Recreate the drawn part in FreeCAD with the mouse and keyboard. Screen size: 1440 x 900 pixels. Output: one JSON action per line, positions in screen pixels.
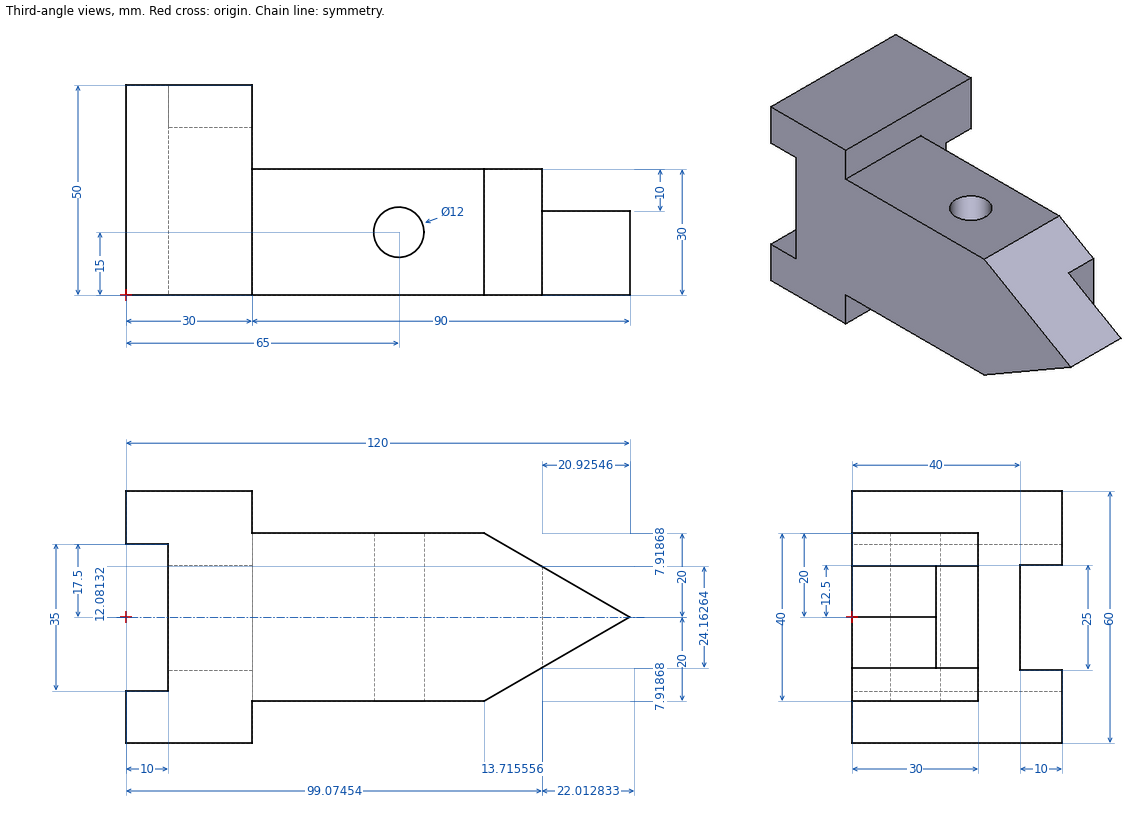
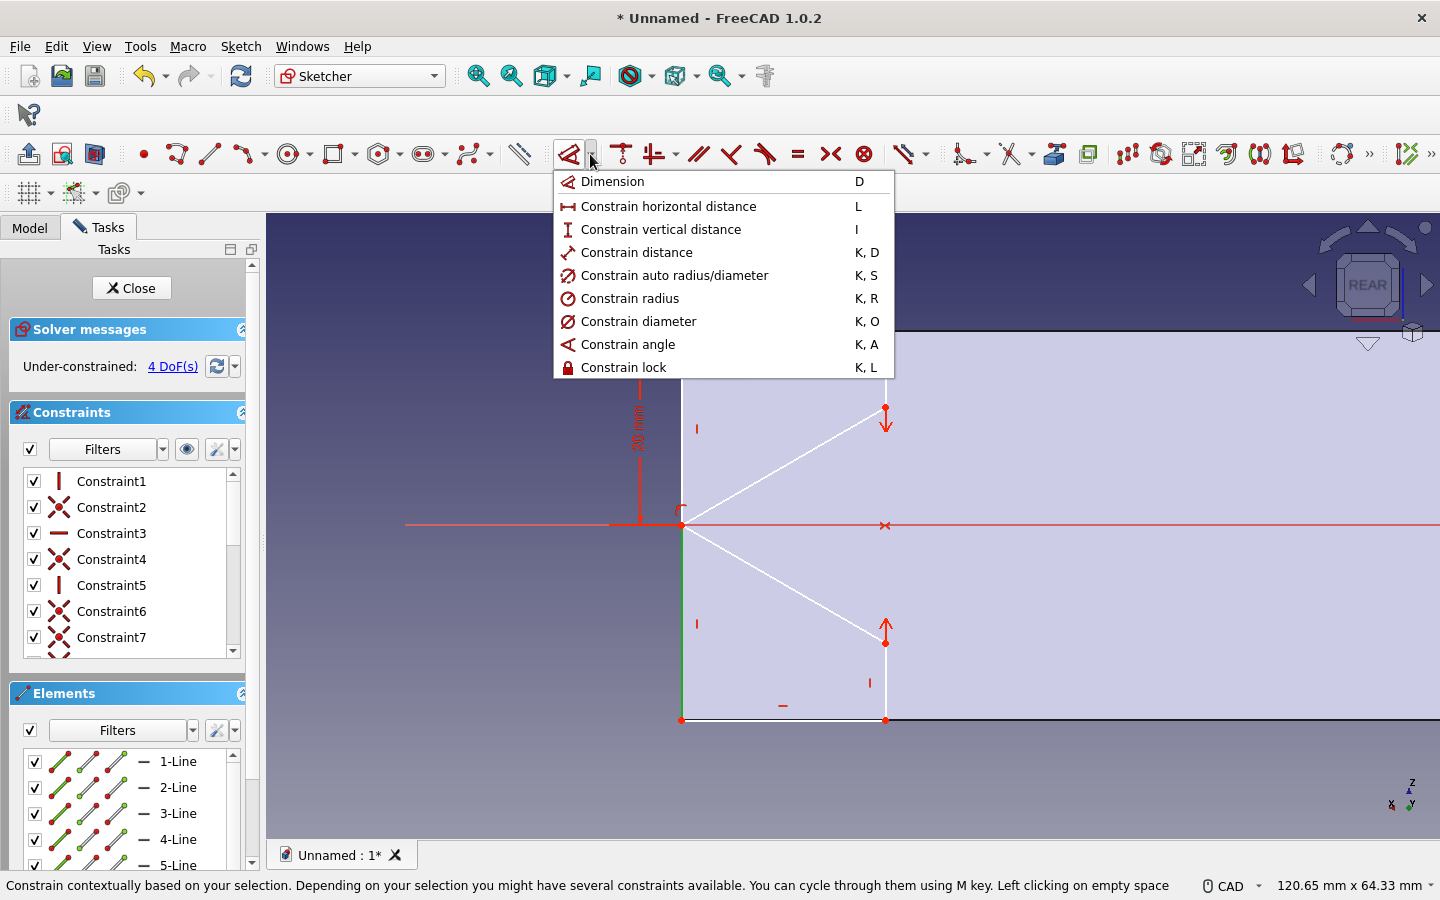
{"action": "left_click", "coordinate": [724, 230]}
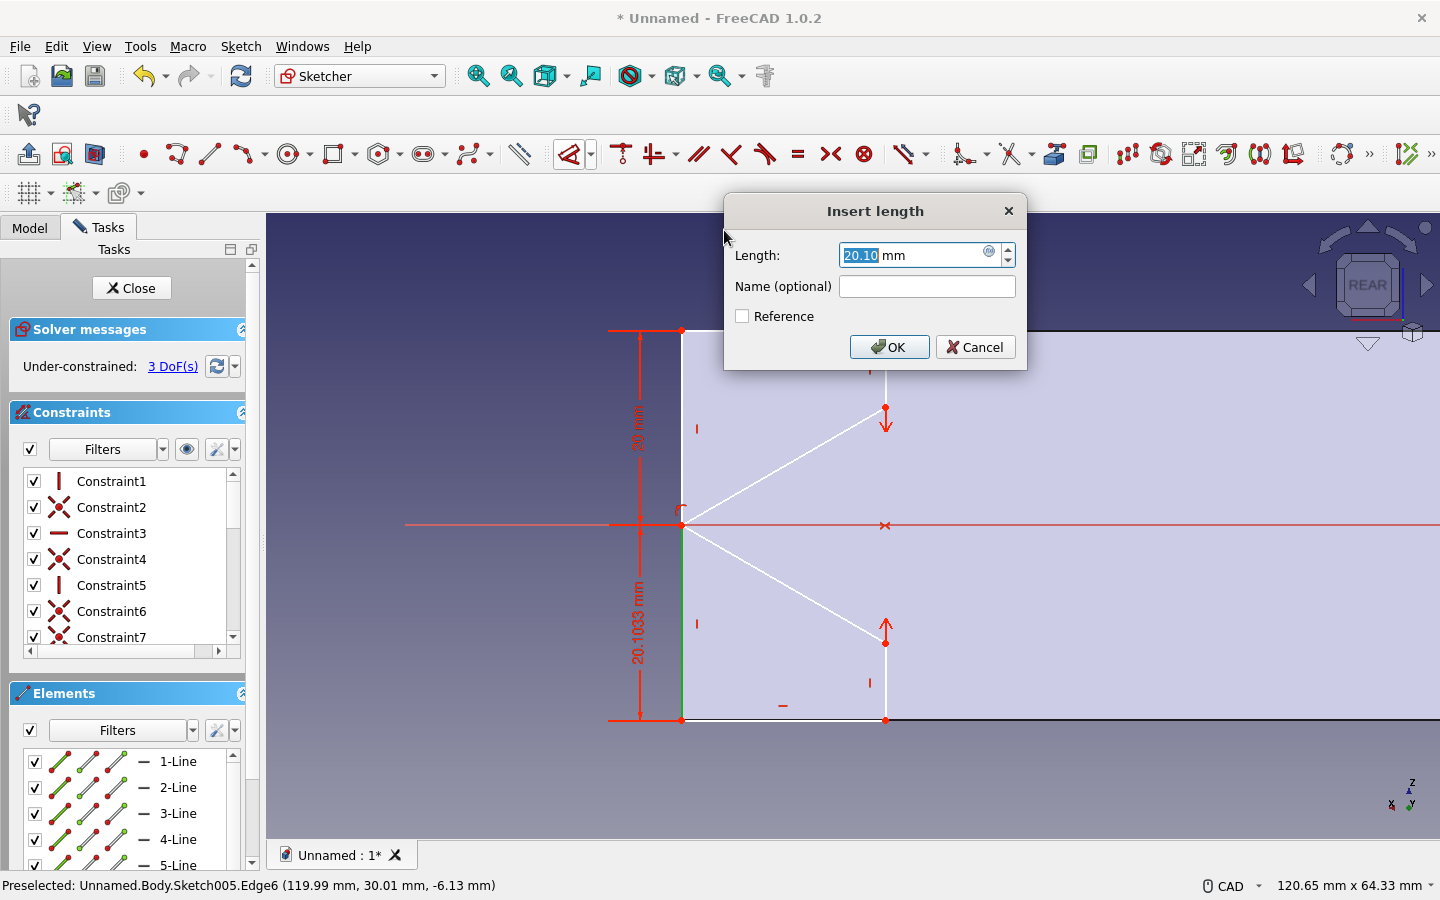
{"action": "type", "text": "20"}
{"action": "key", "text": "Return"}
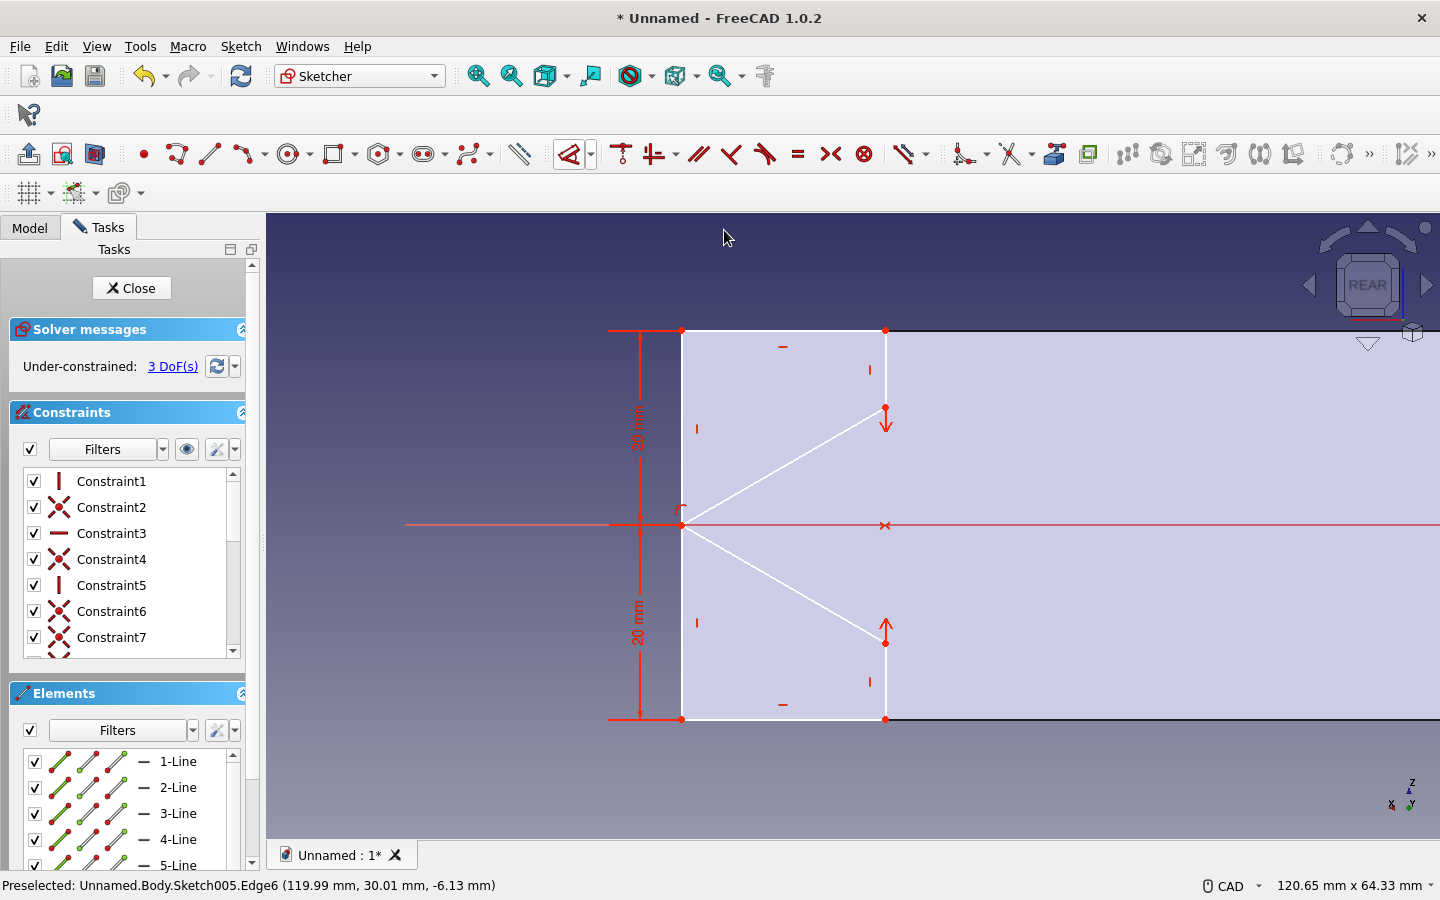
{"action": "left_click", "coordinate": [682, 331]}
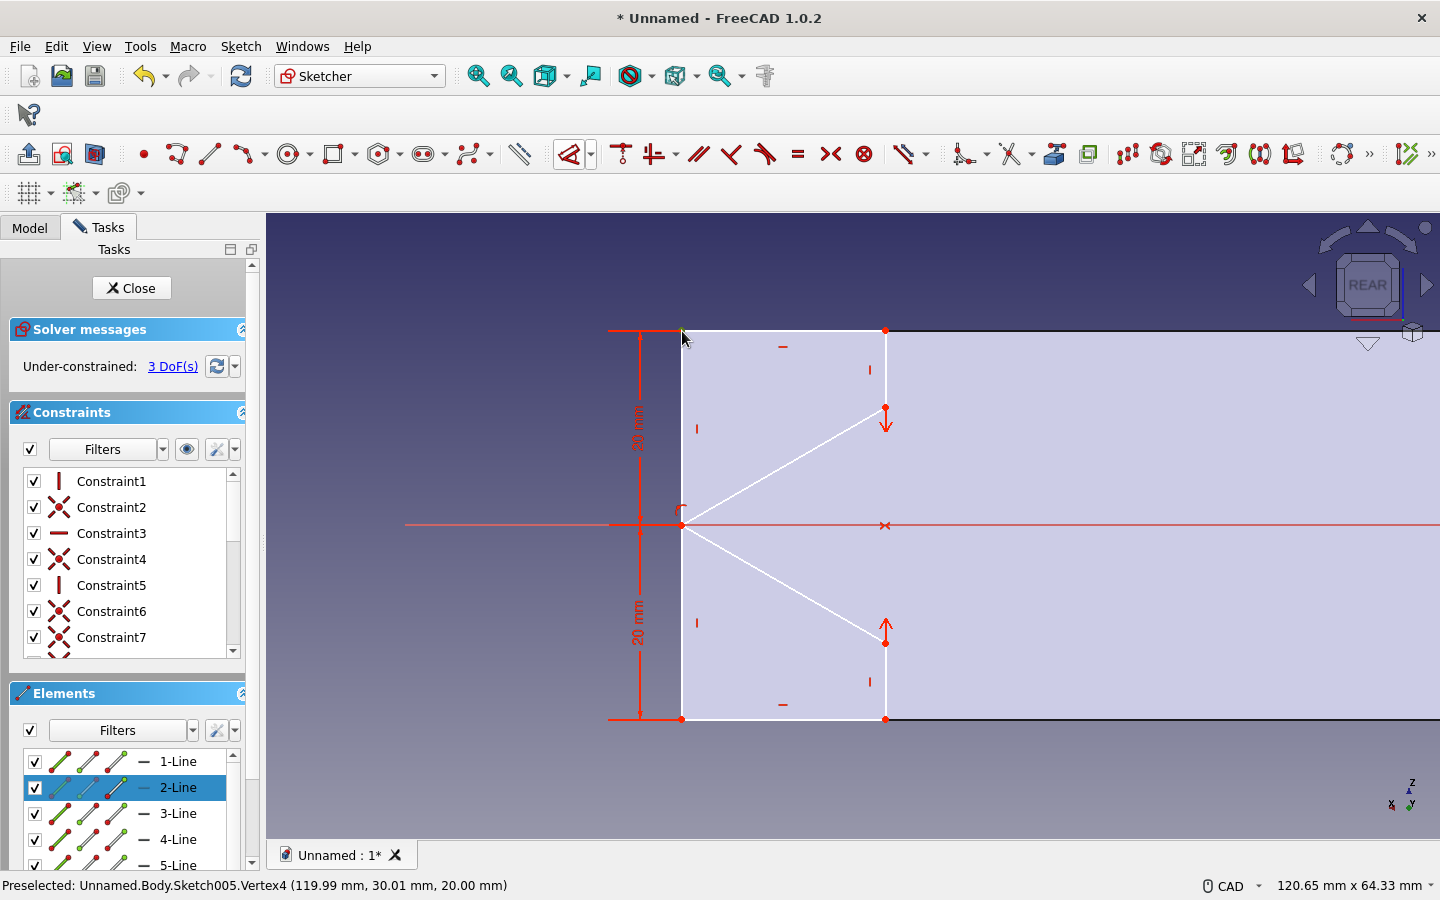
{"action": "left_click", "coordinate": [590, 154]}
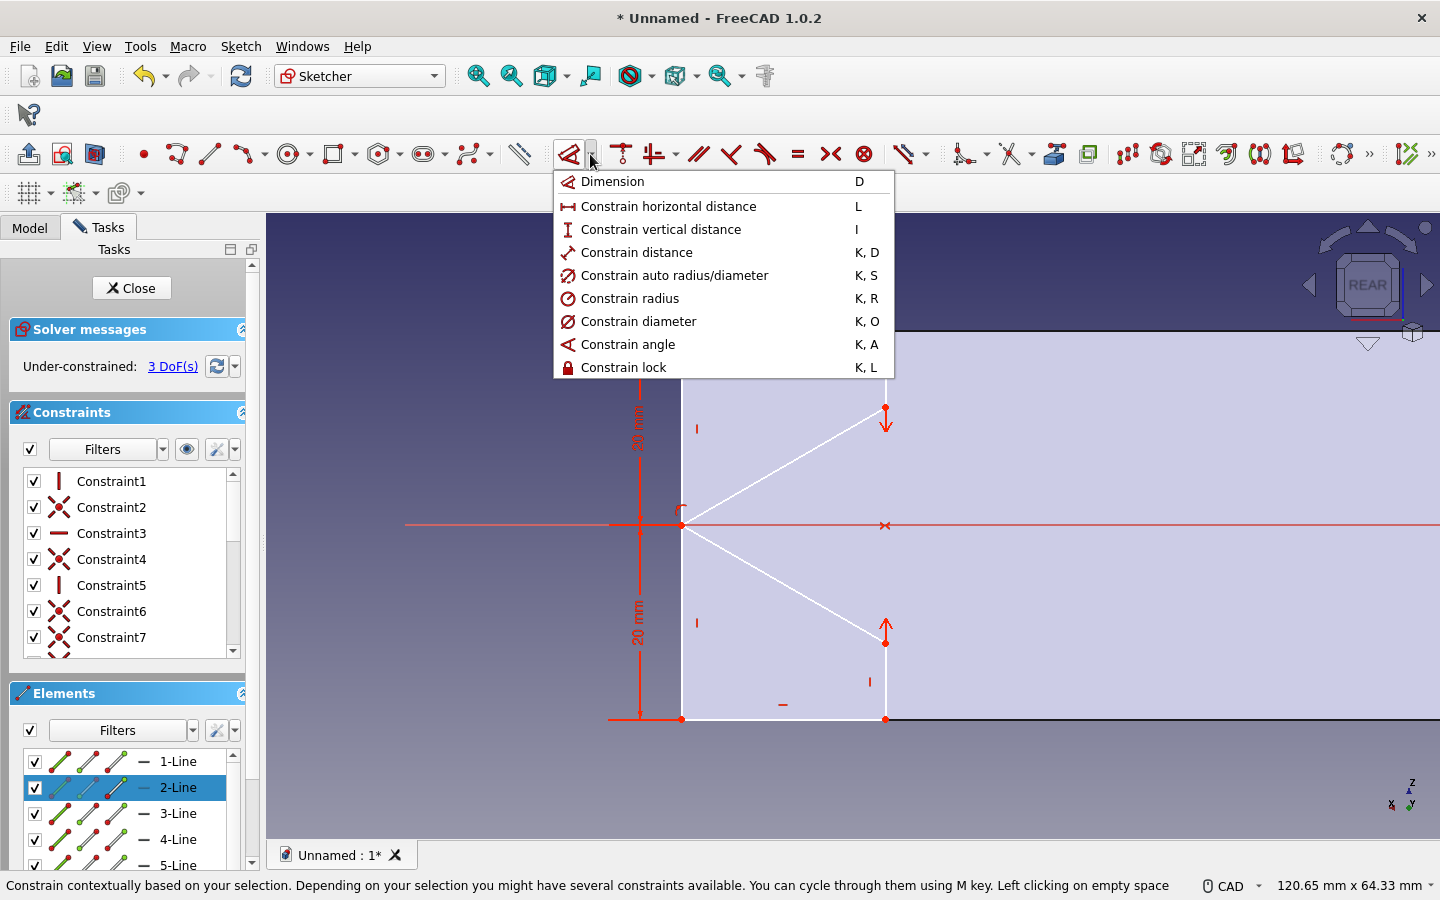
{"action": "left_click", "coordinate": [724, 206]}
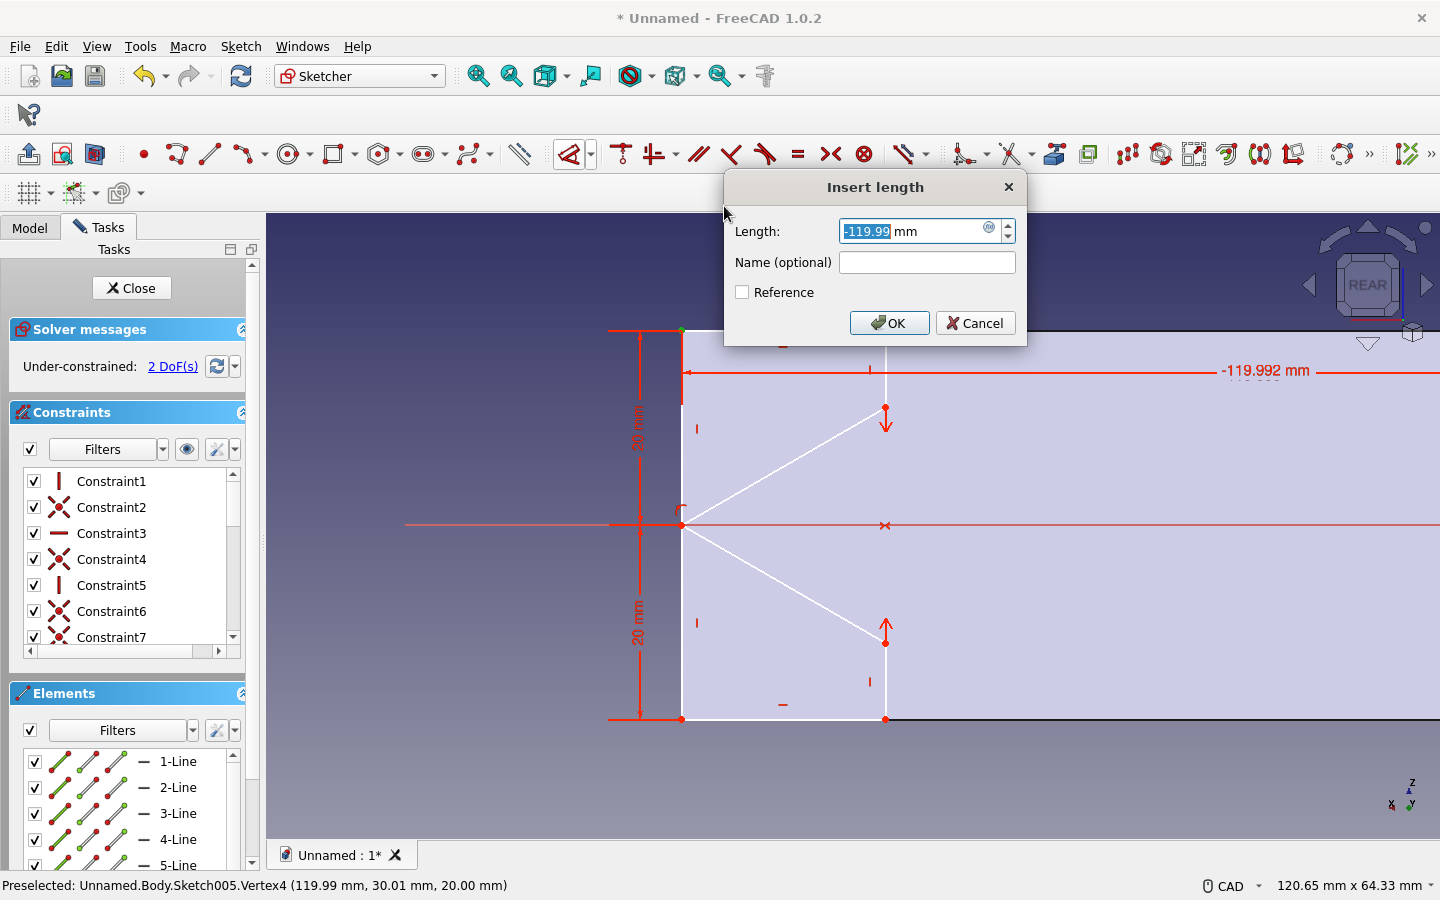
{"action": "type", "text": "-120"}
{"action": "key", "text": "Return"}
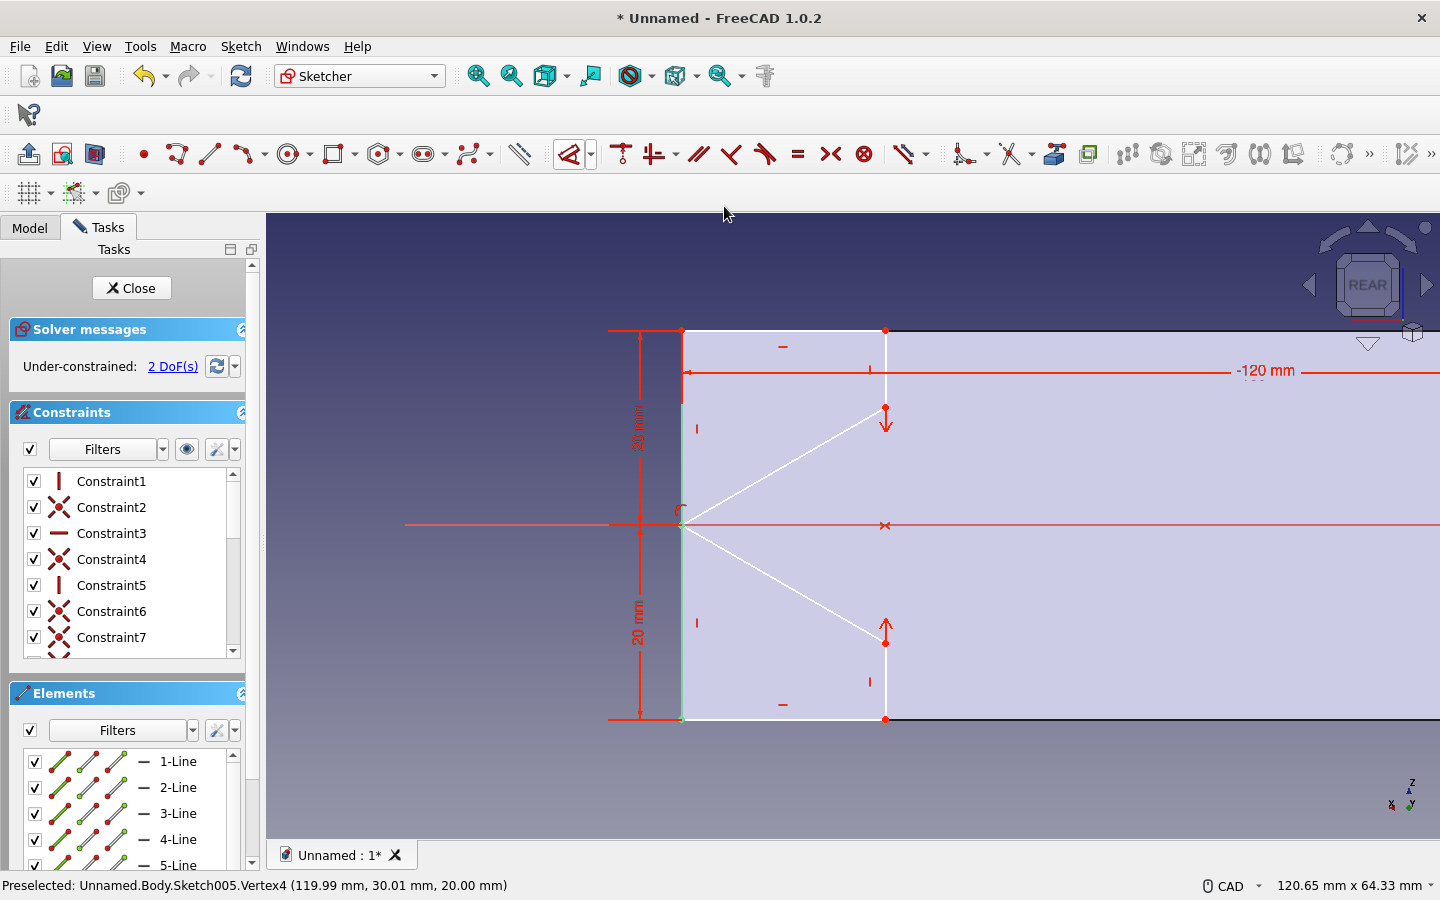
{"action": "left_click", "coordinate": [886, 384]}